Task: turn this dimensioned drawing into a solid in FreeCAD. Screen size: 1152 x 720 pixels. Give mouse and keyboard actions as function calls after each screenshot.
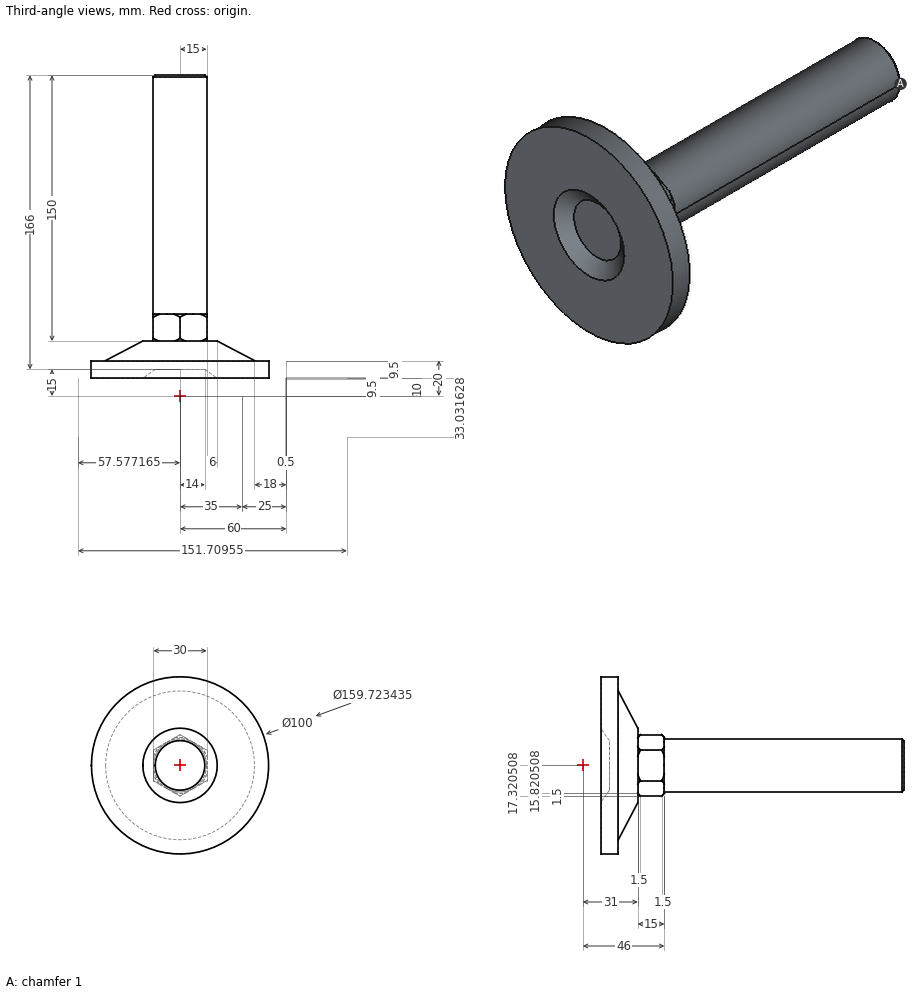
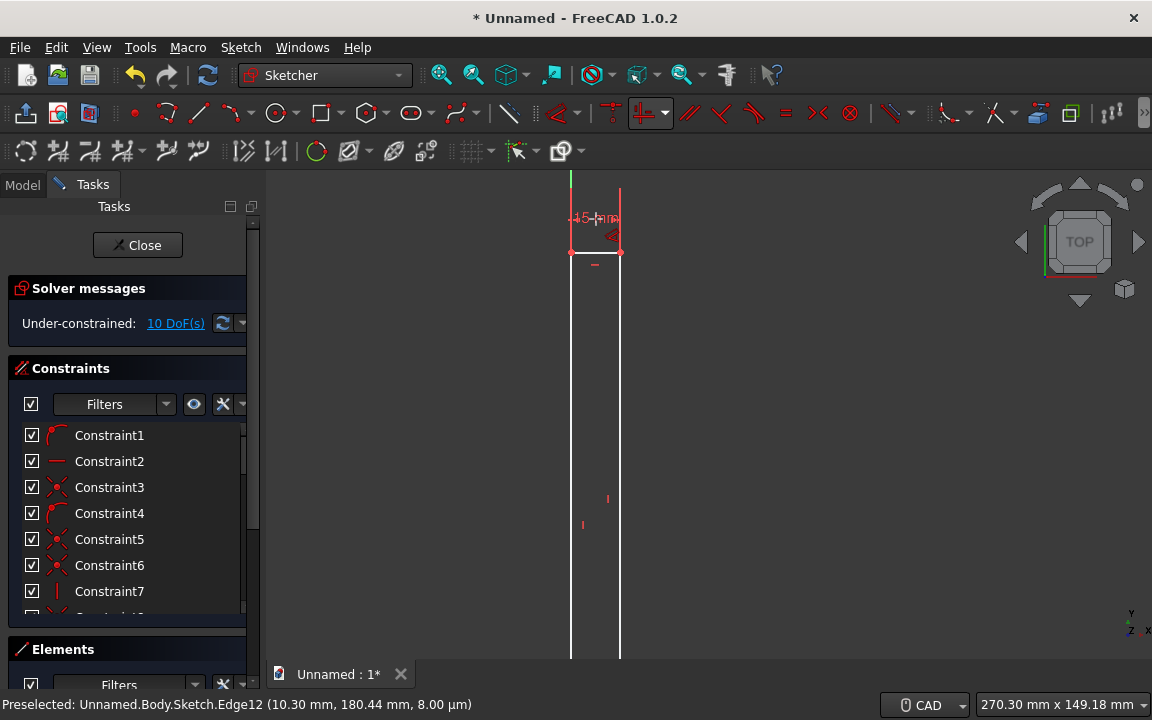
scroll(605, 253, down, 3)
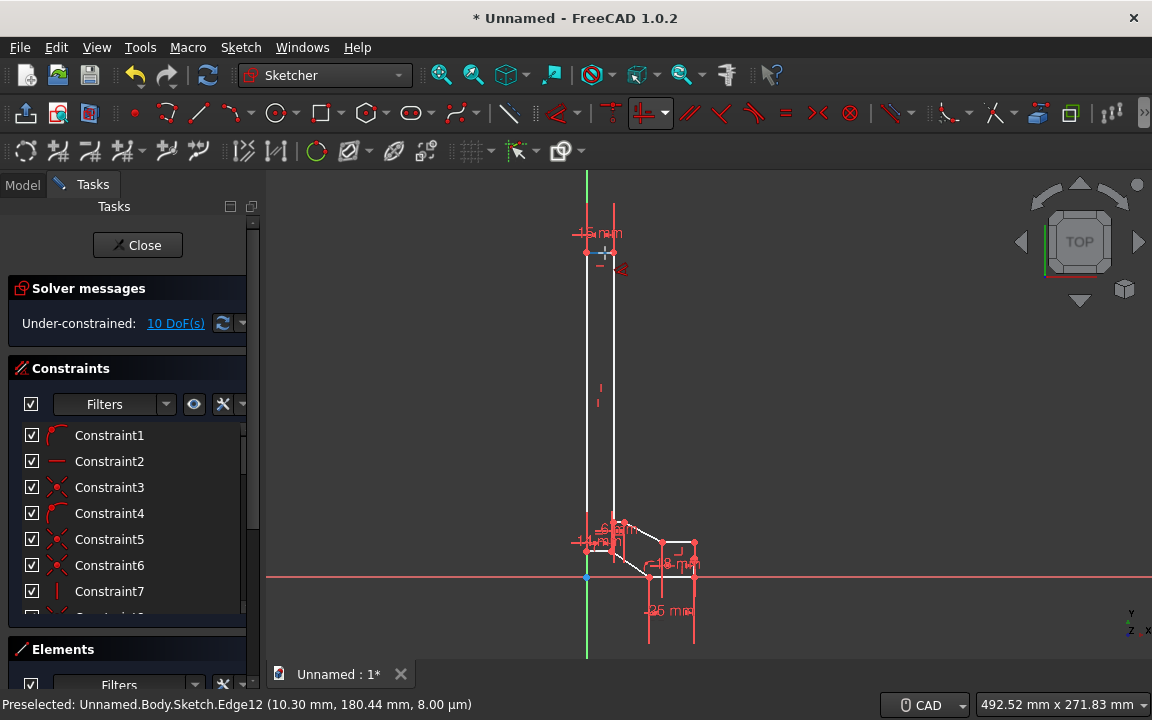
scroll(694, 571, up, 5)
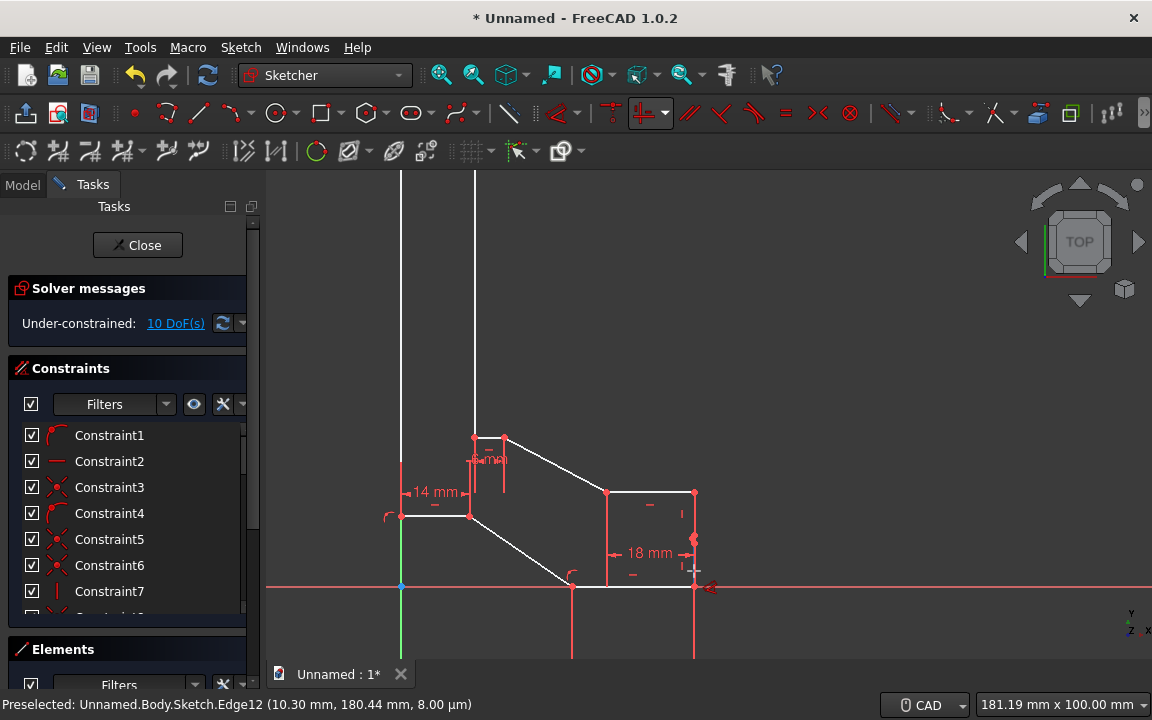
click(694, 570)
click(728, 565)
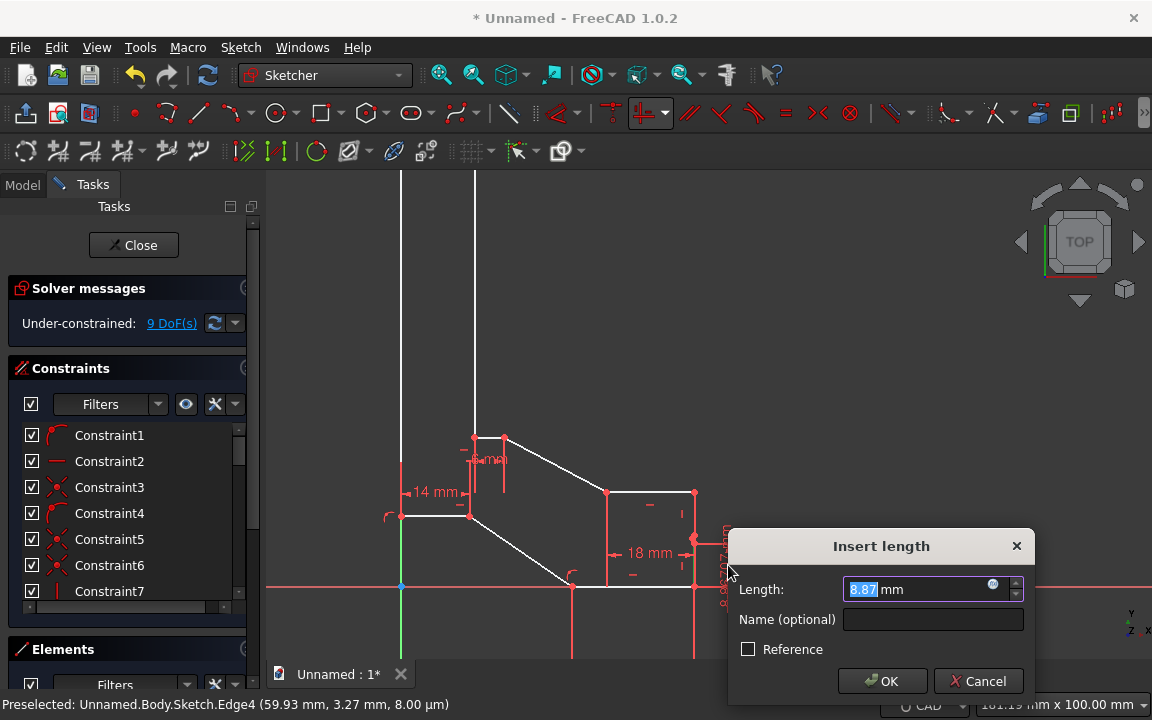
text(9.5)
key(Return)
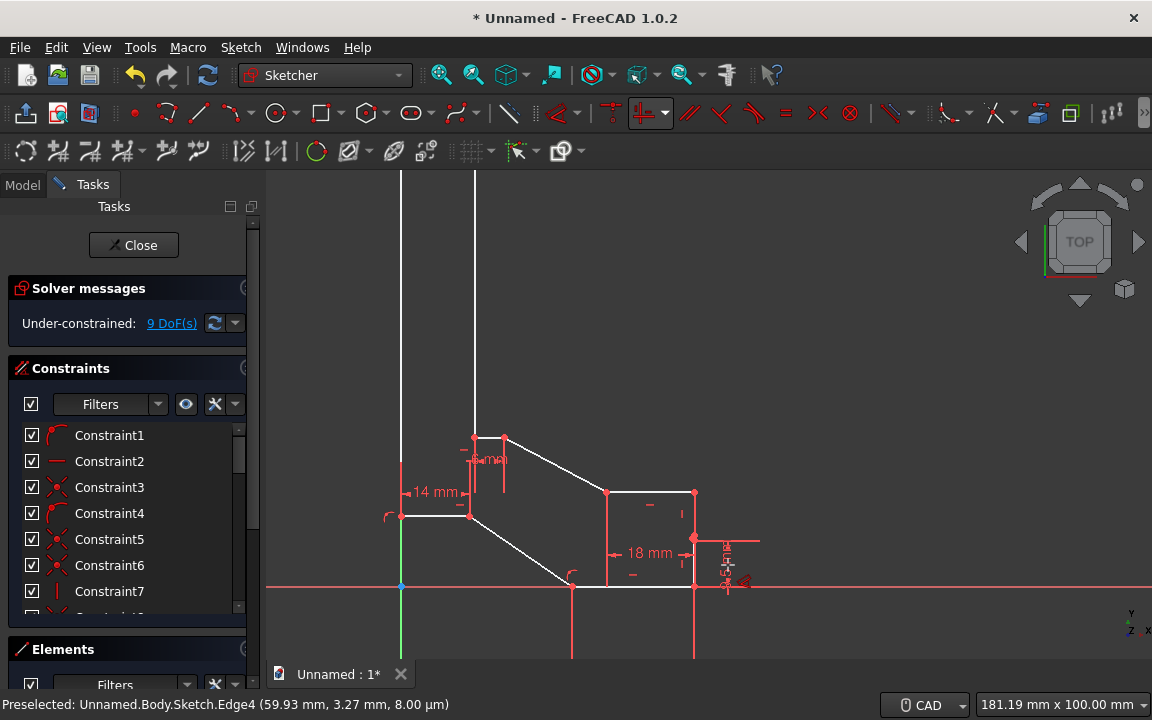
click(695, 523)
click(729, 514)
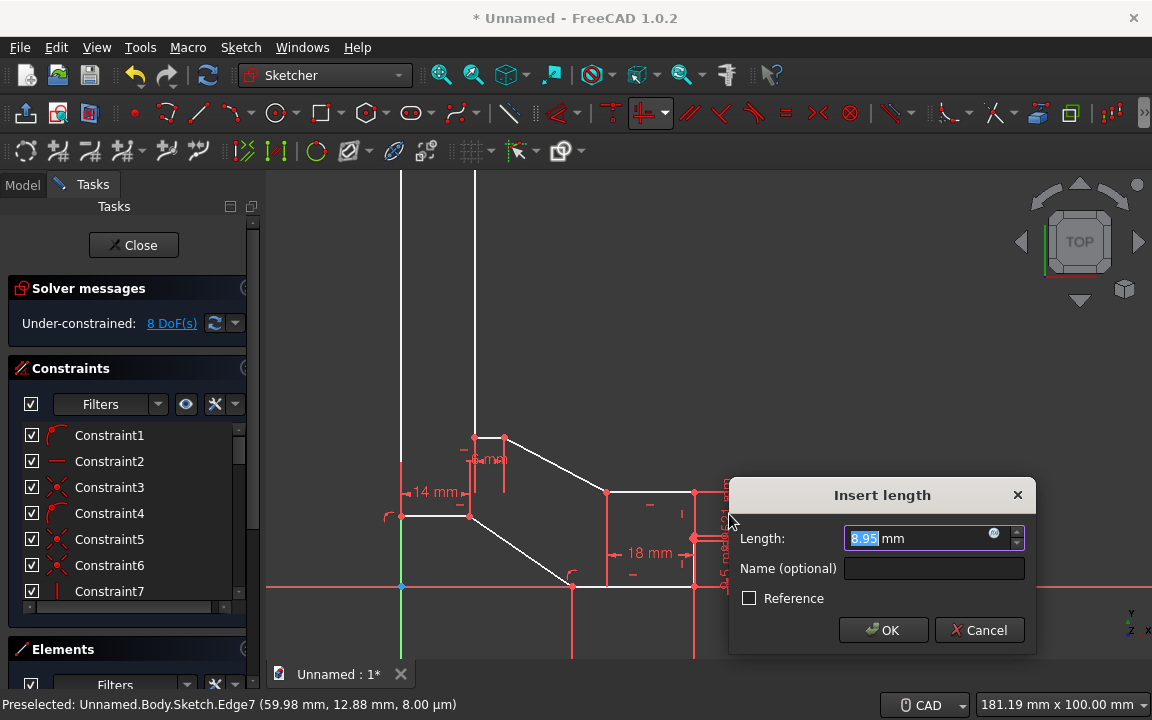
text(9.5)
key(Return)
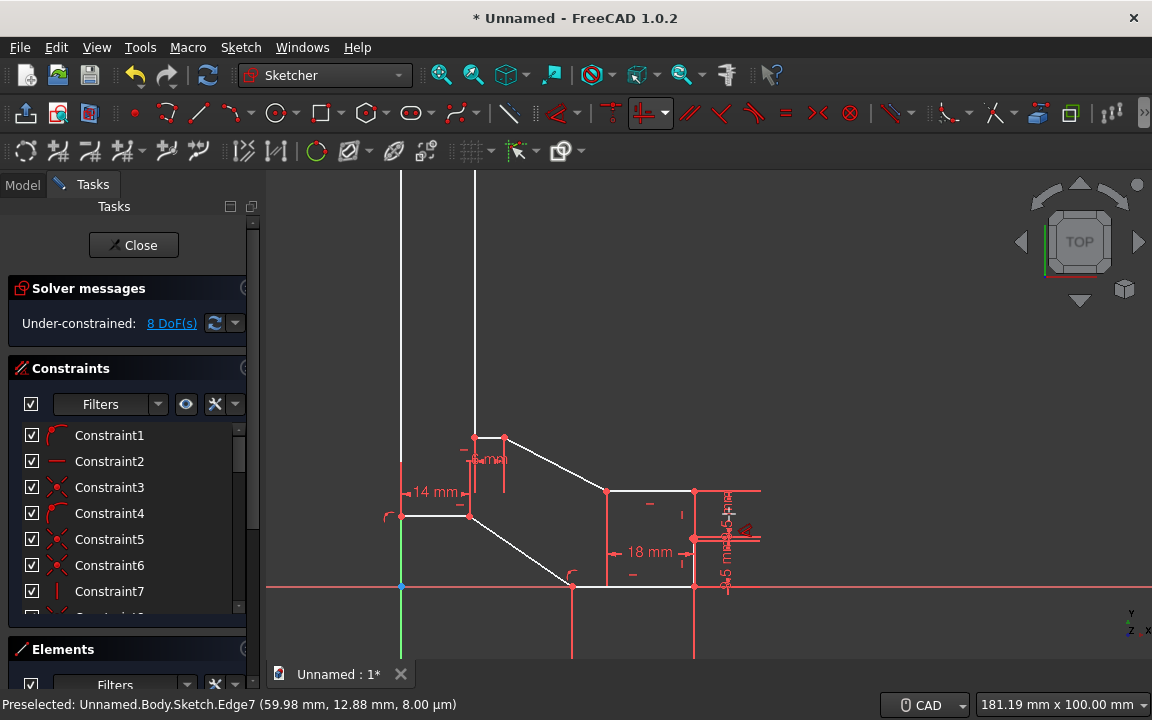
click(475, 218)
click(441, 318)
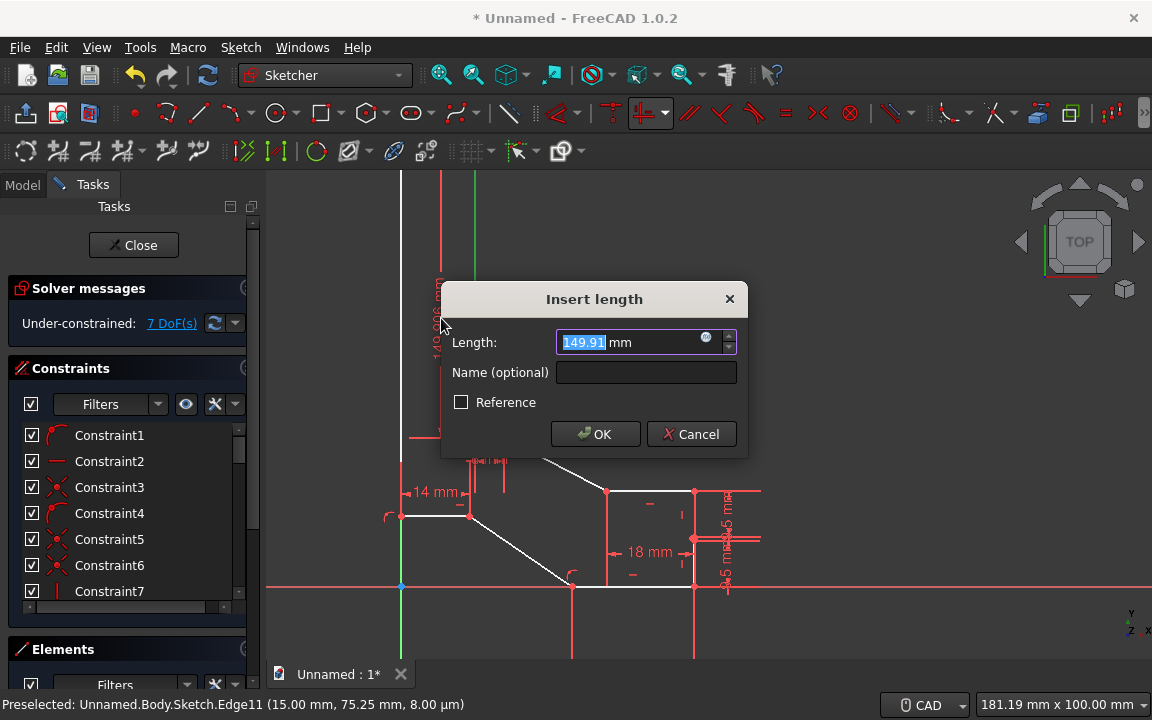
text(150)
key(Return)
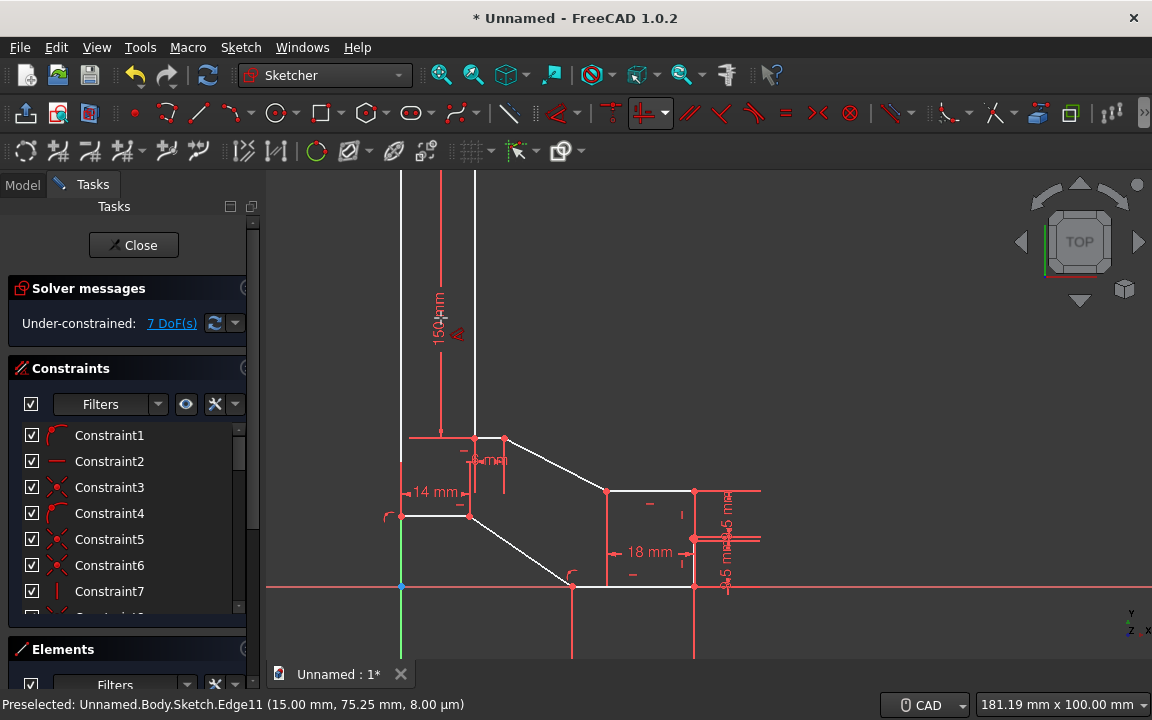
click(401, 273)
click(367, 357)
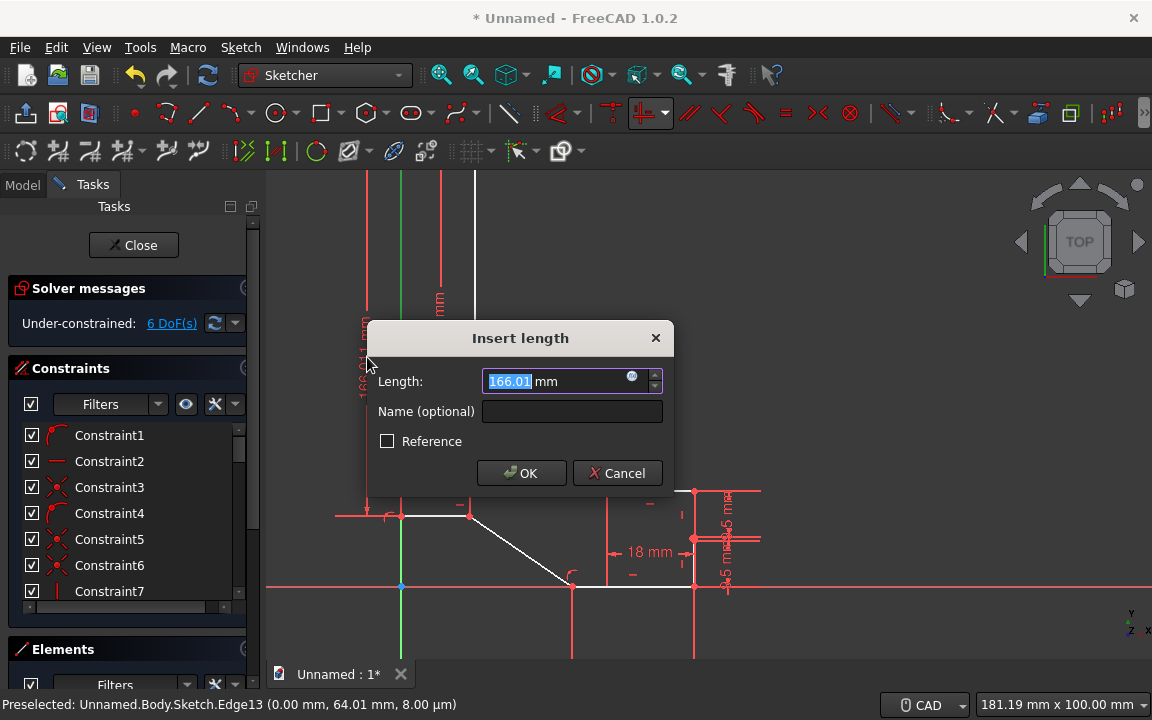
text(166)
key(Return)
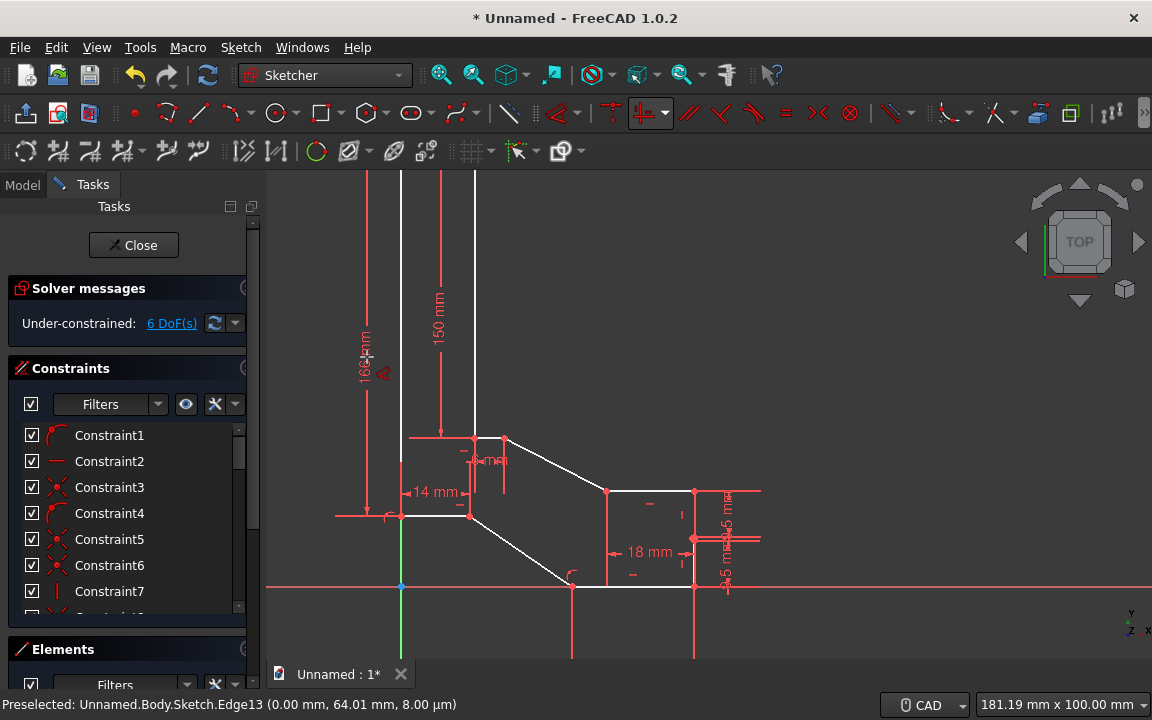
click(401, 516)
click(367, 552)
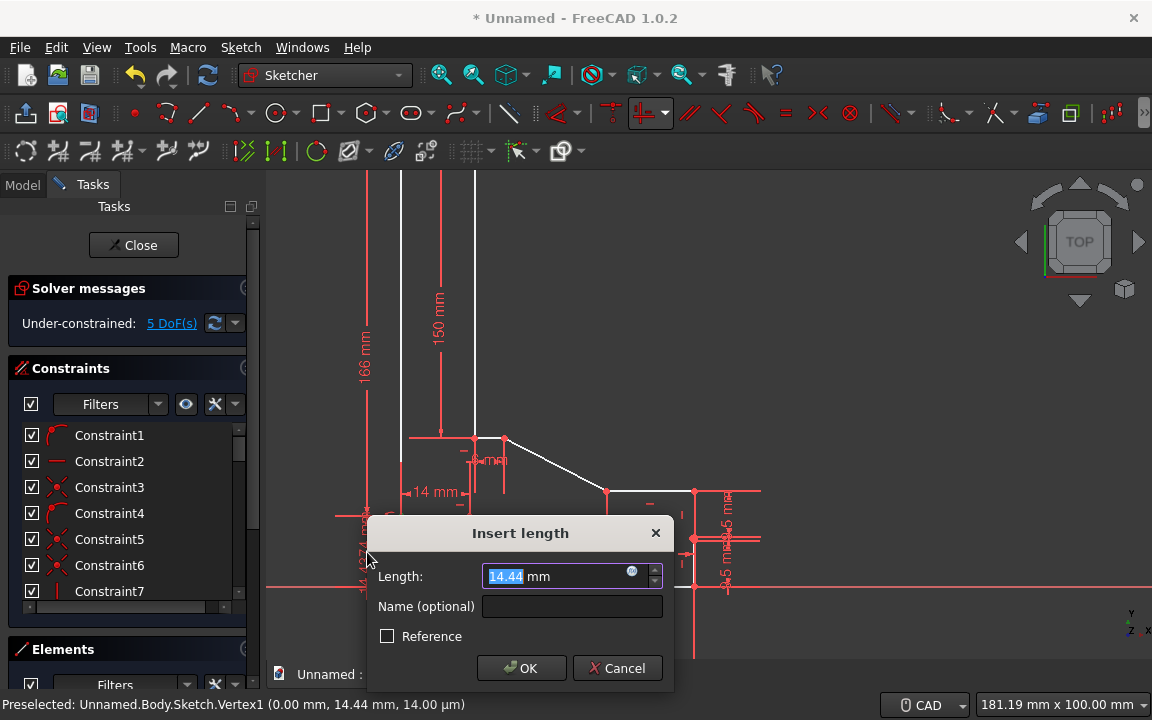
text(15)
key(Return)